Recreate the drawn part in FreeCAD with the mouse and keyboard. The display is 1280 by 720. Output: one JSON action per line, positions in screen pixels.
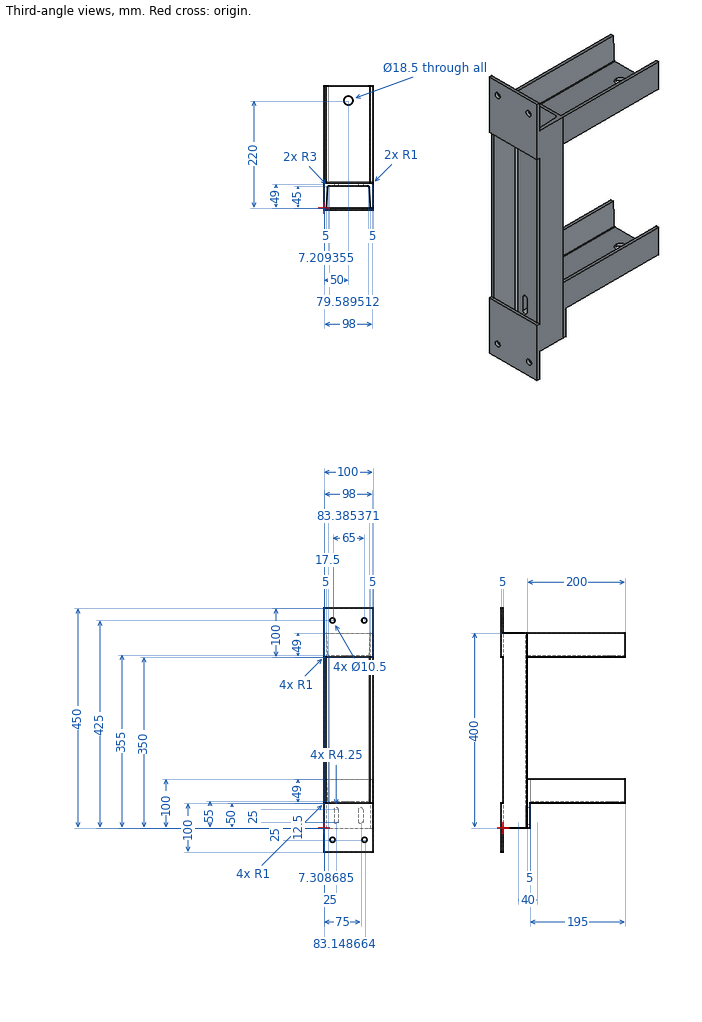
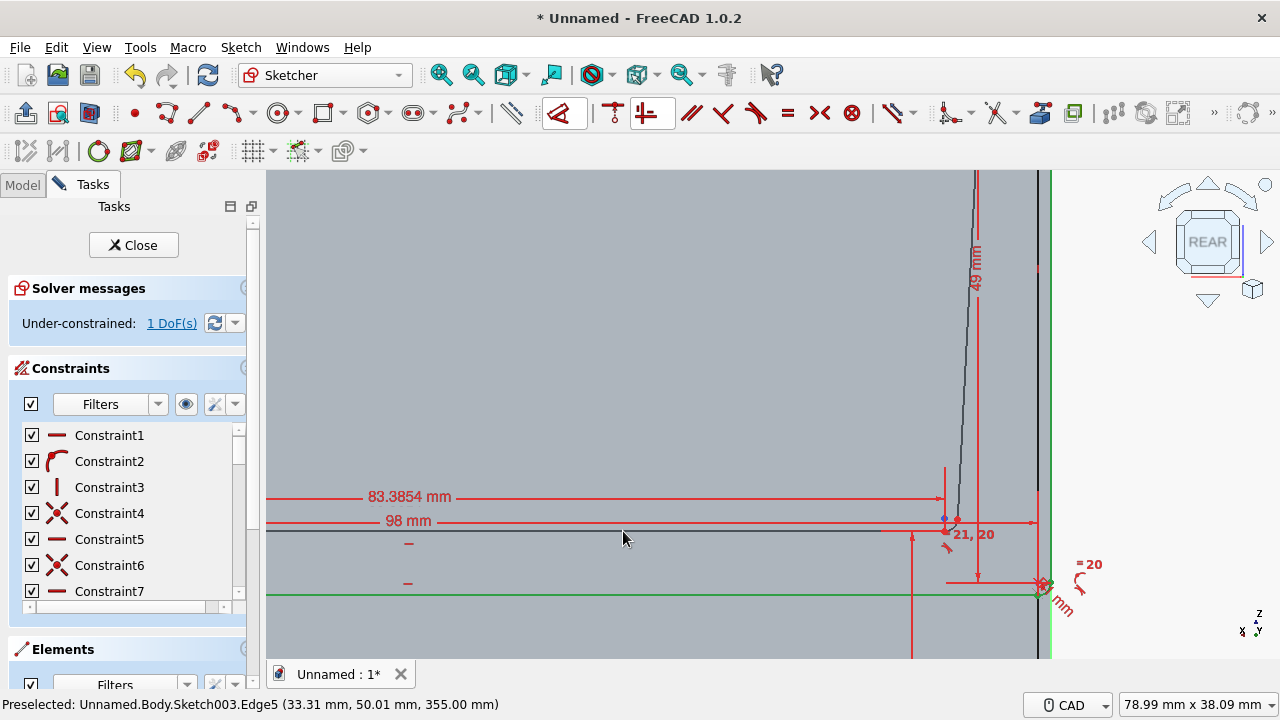
{"action": "left_click", "coordinate": [958, 519]}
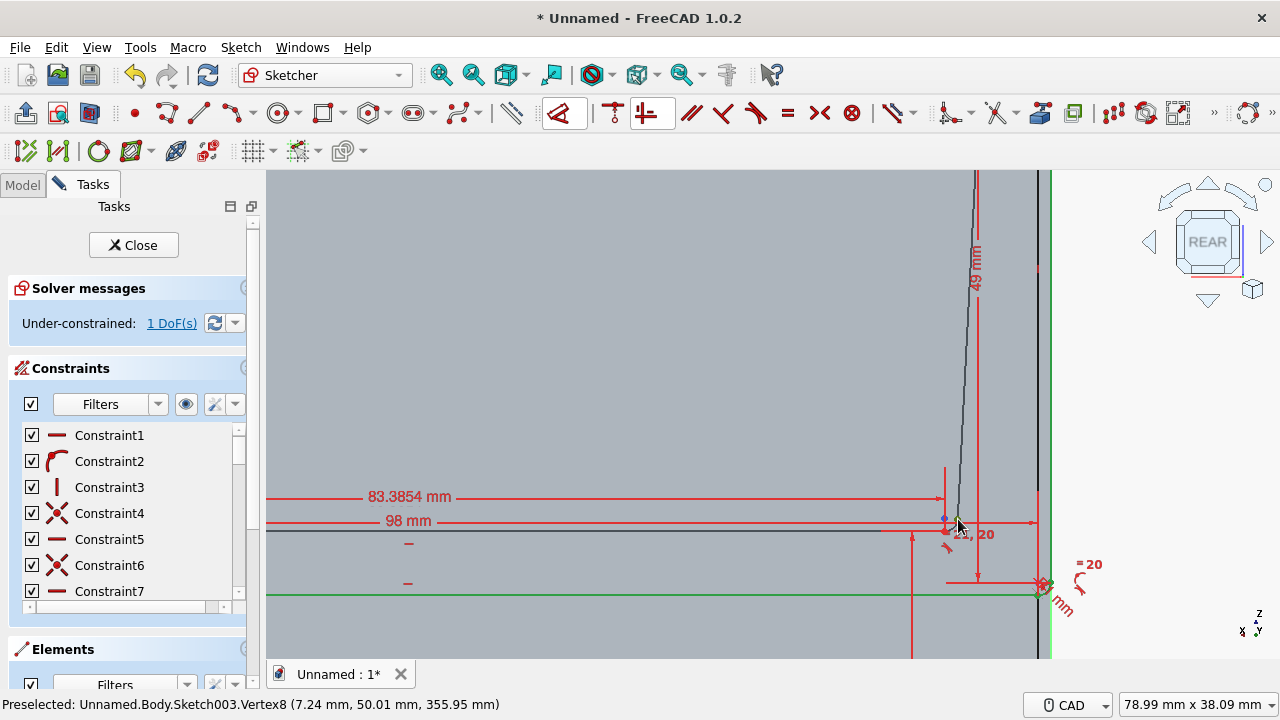
{"action": "left_click", "coordinate": [582, 114]}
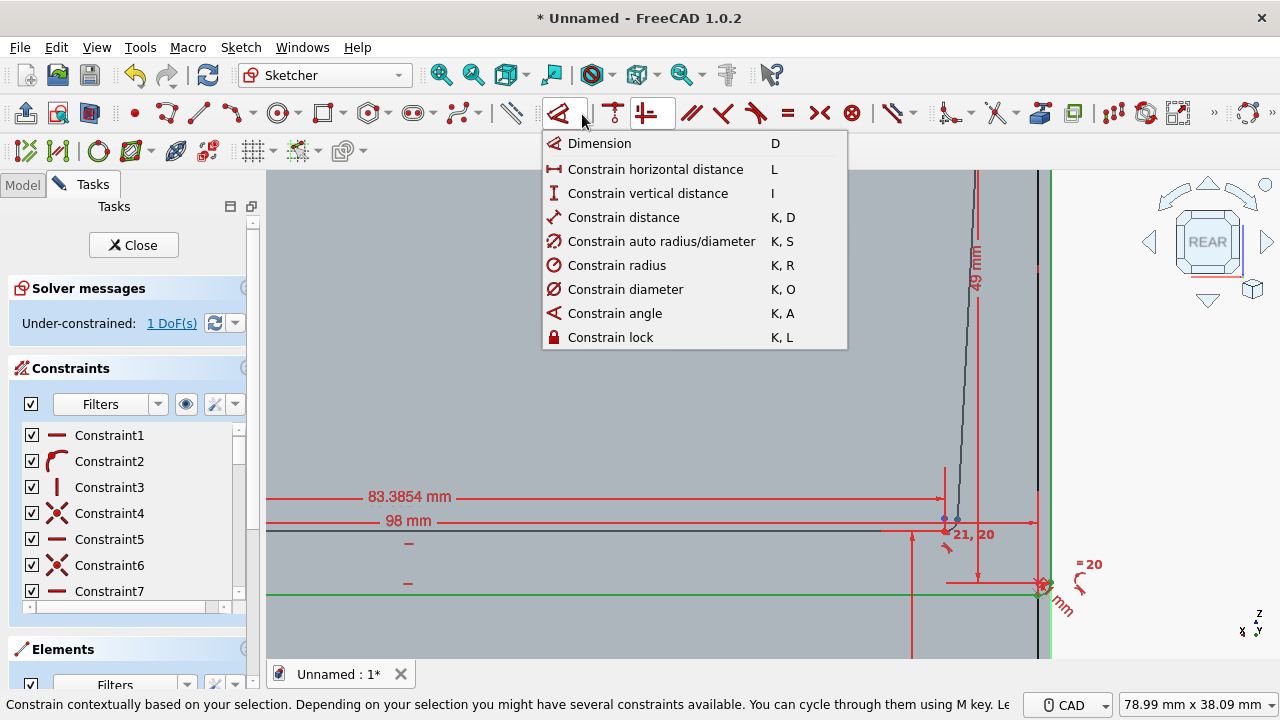
{"action": "left_click", "coordinate": [695, 169]}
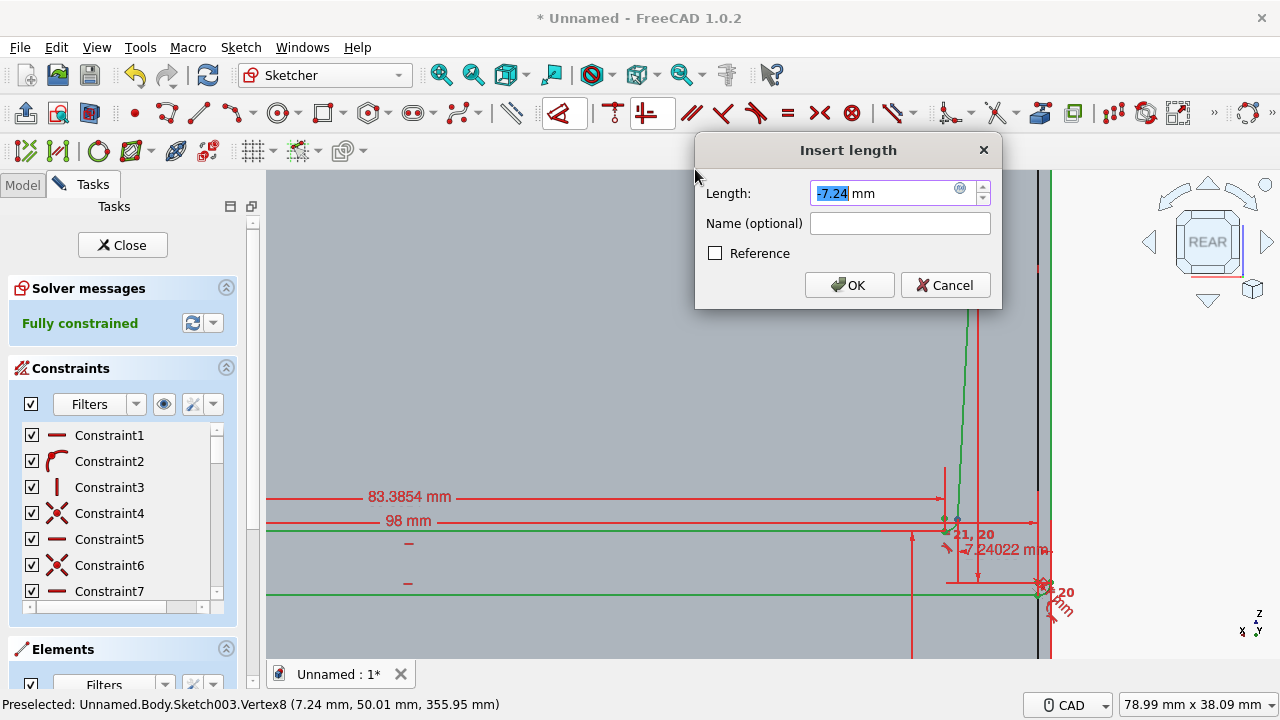
{"action": "type", "text": "-7.308685"}
{"action": "key", "text": "Return"}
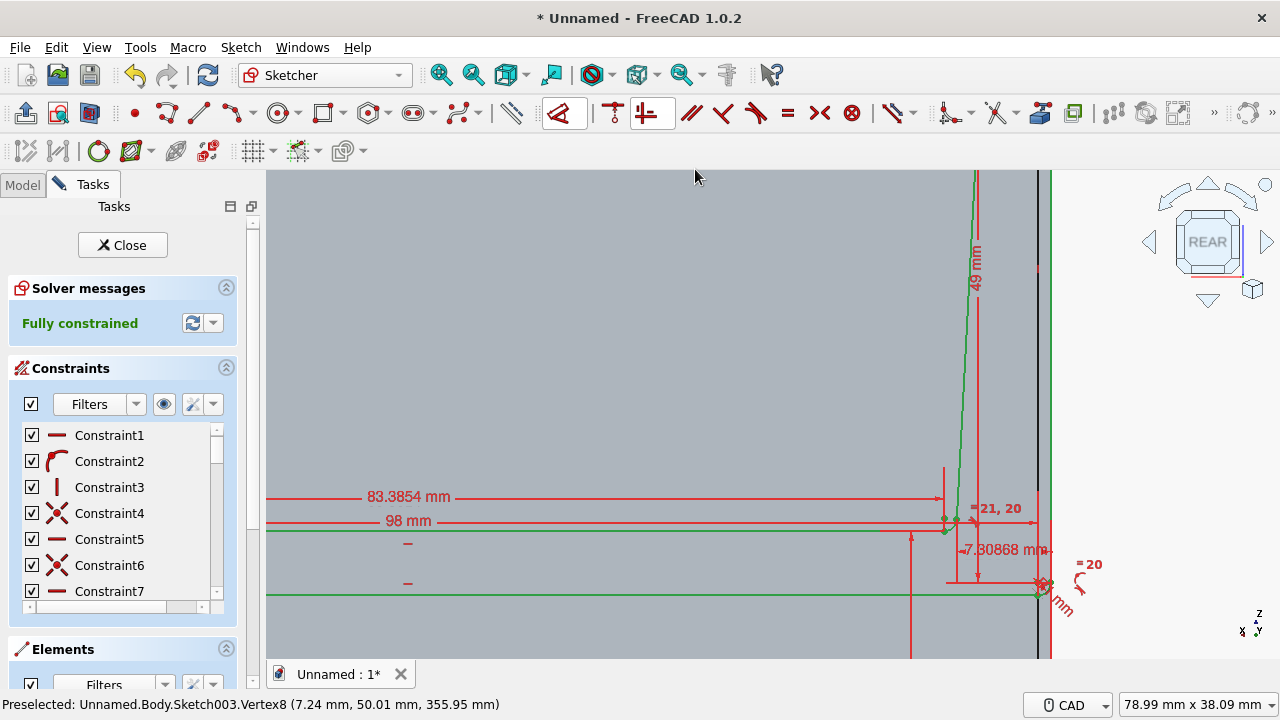
{"action": "left_click", "coordinate": [123, 245]}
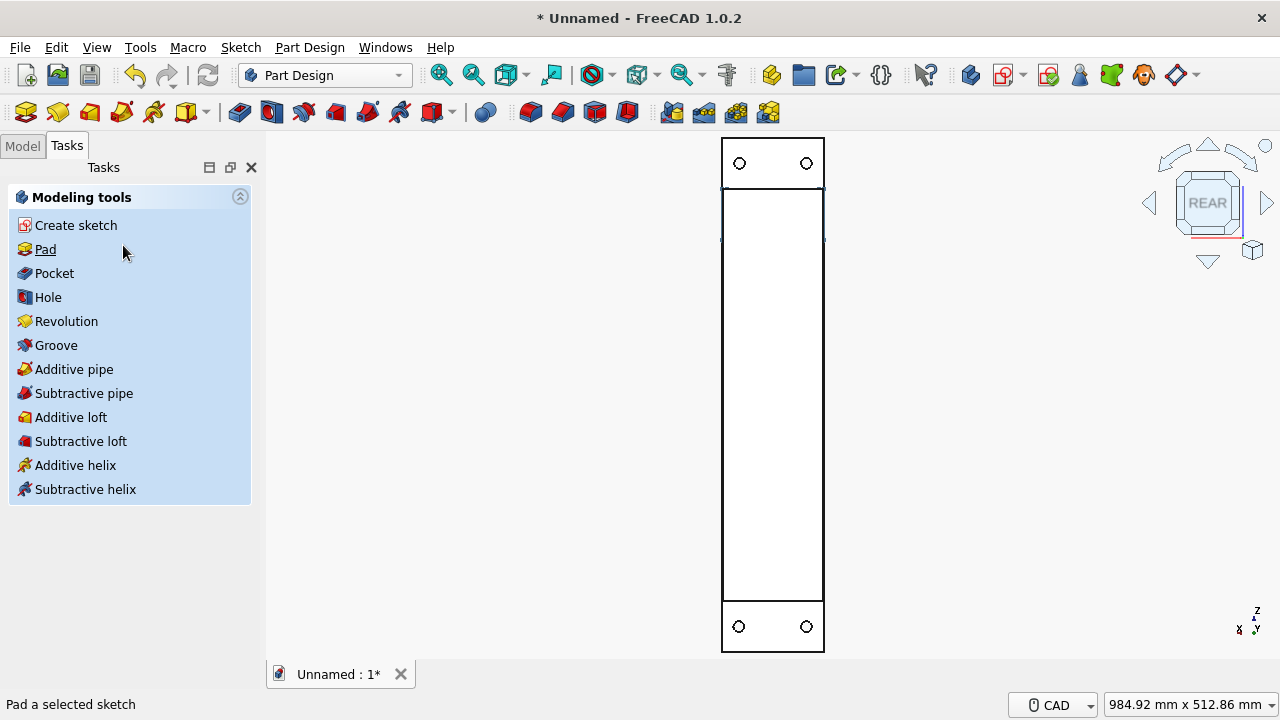
{"action": "left_click", "coordinate": [26, 112]}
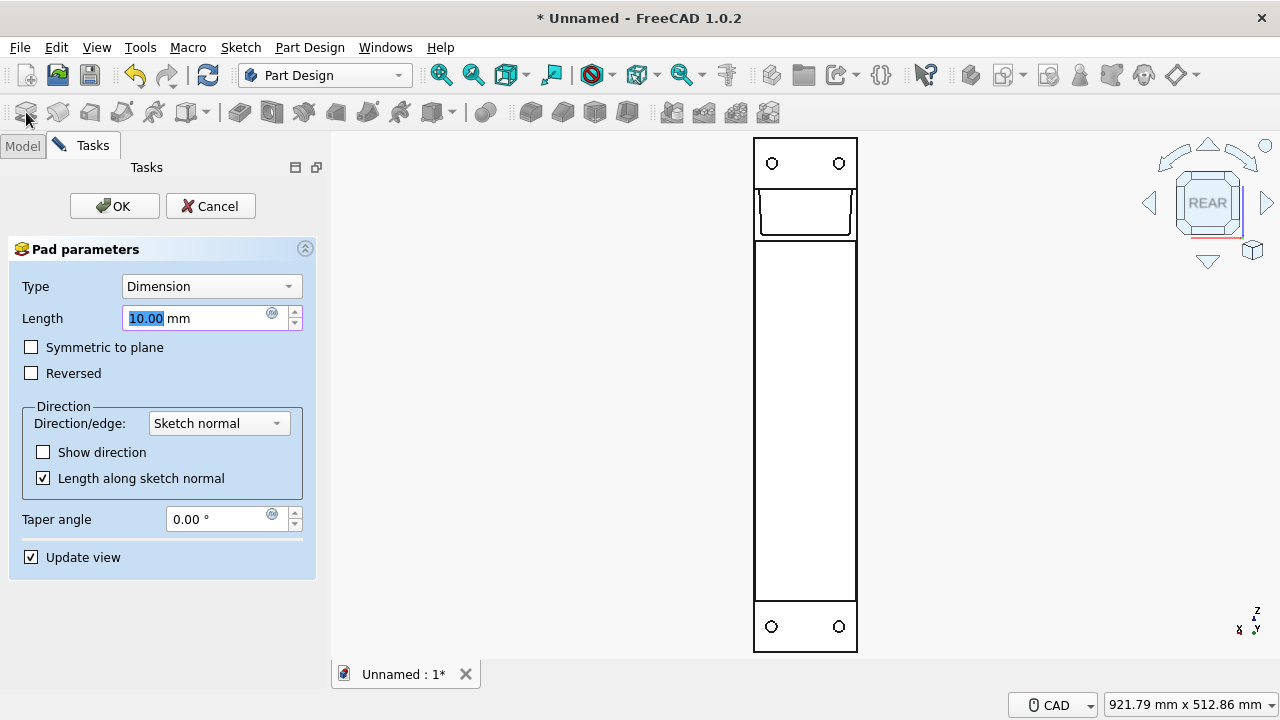
{"action": "type", "text": "200"}
{"action": "key", "text": "Tab"}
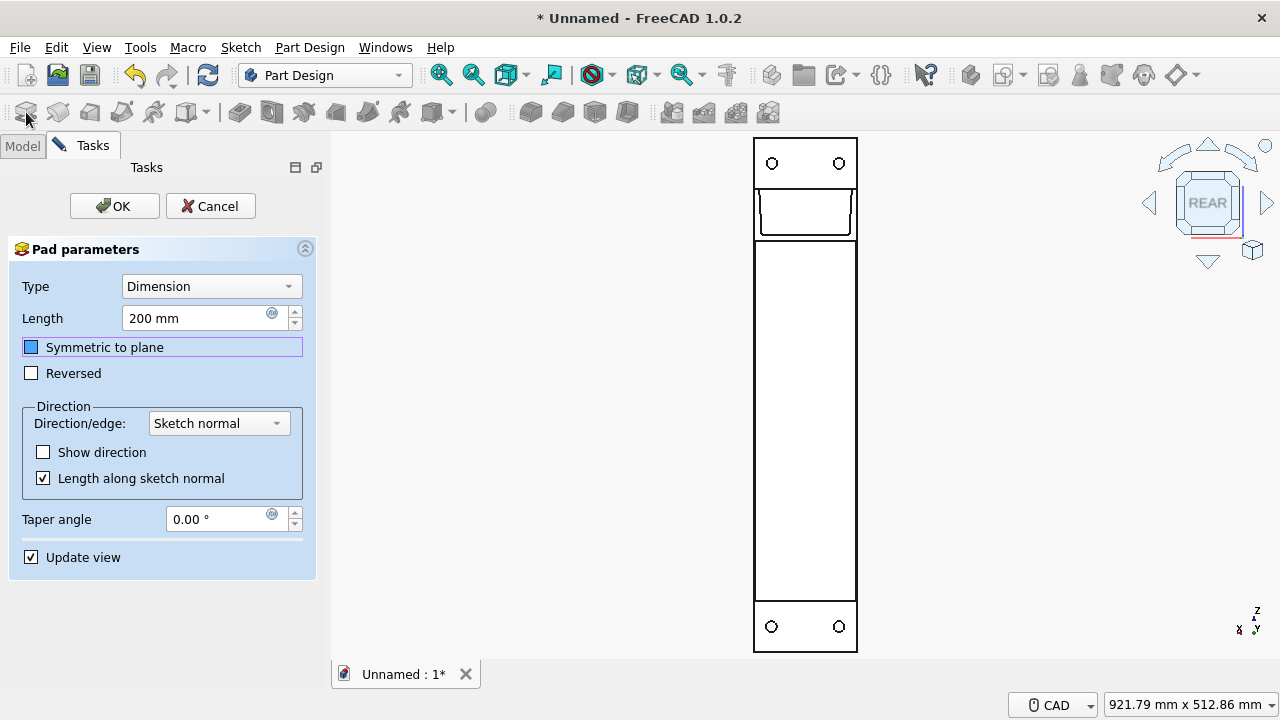
{"action": "left_click", "coordinate": [115, 206]}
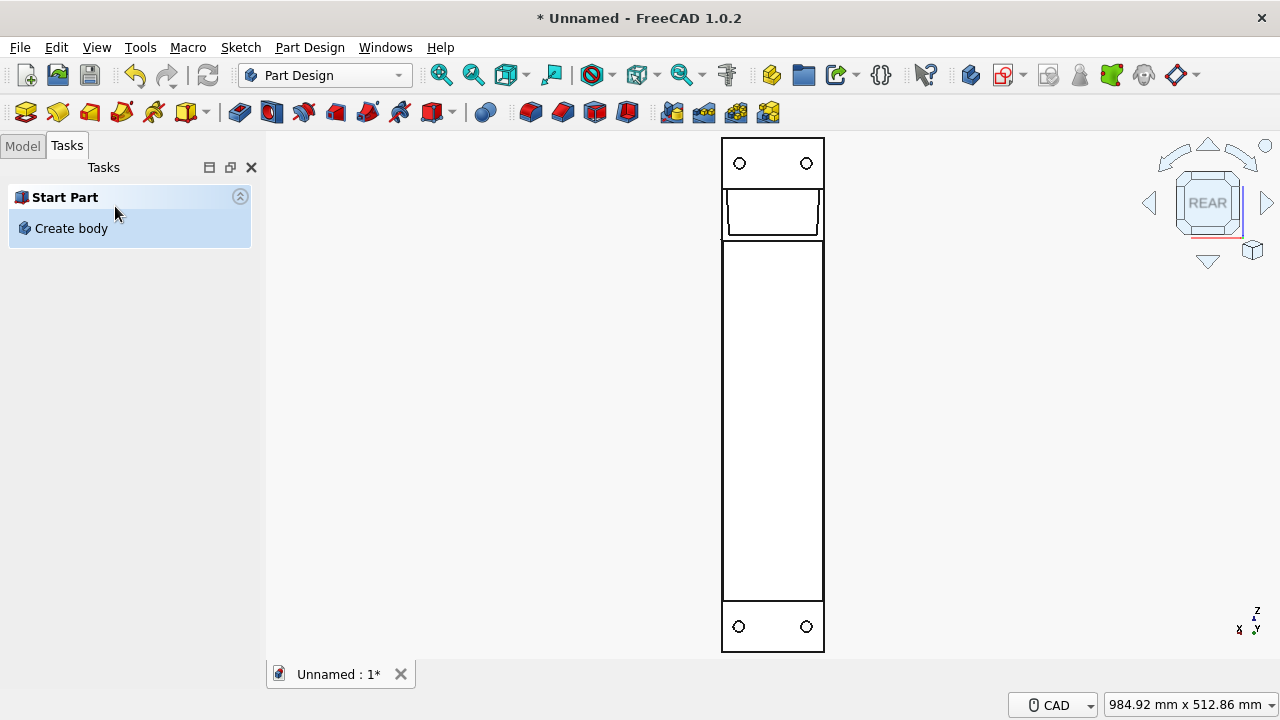
{"action": "left_click", "coordinate": [773, 317]}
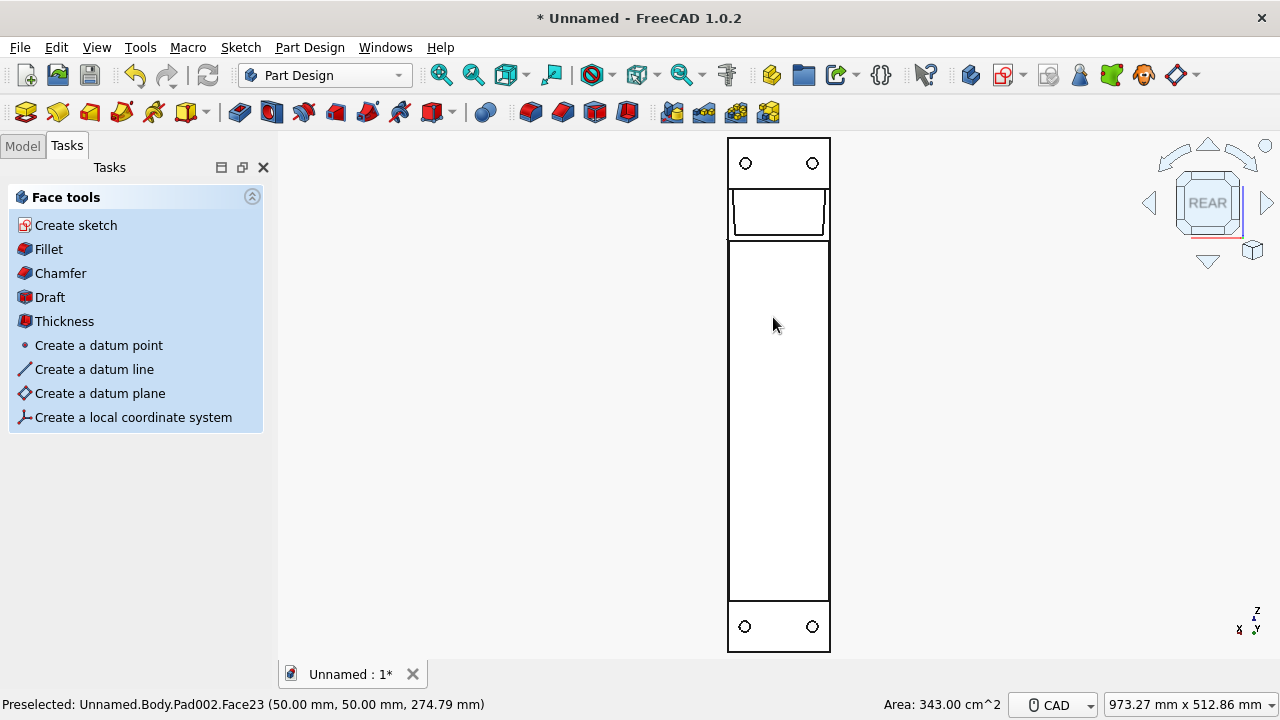
{"action": "left_click", "coordinate": [1004, 76]}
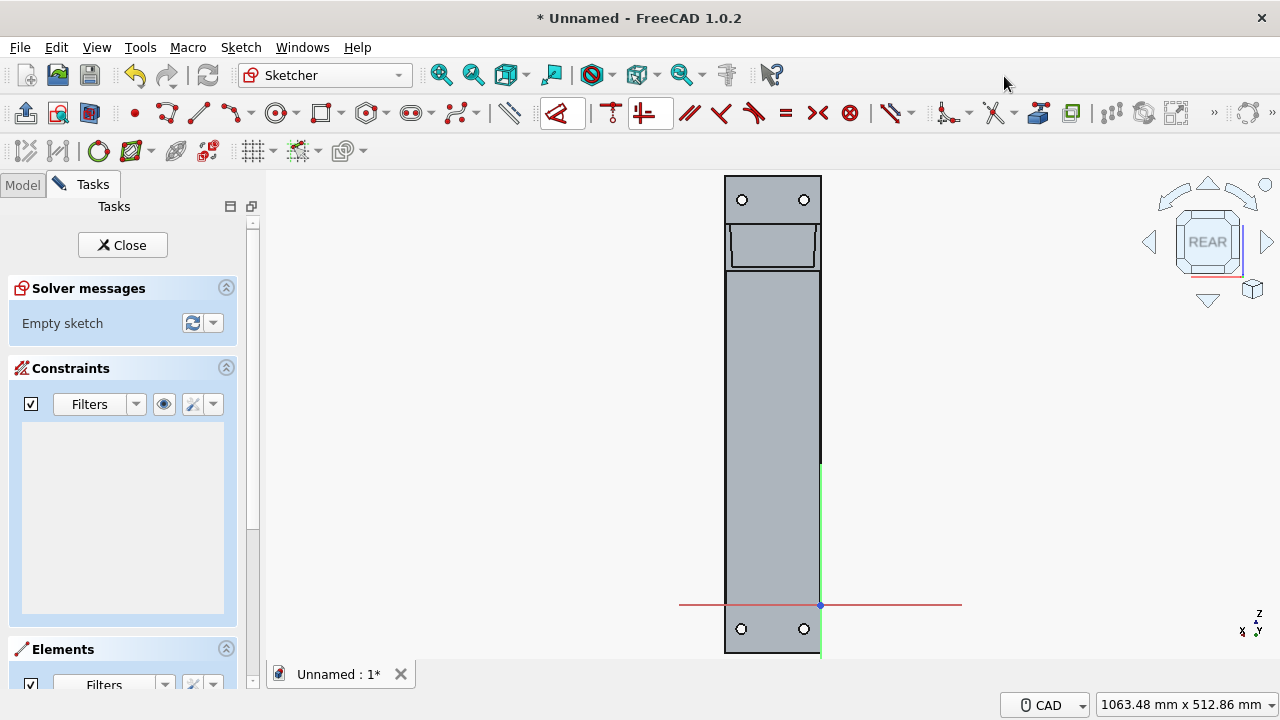
{"action": "scroll", "coordinate": [803, 619], "scroll_direction": "up", "scroll_amount": 6}